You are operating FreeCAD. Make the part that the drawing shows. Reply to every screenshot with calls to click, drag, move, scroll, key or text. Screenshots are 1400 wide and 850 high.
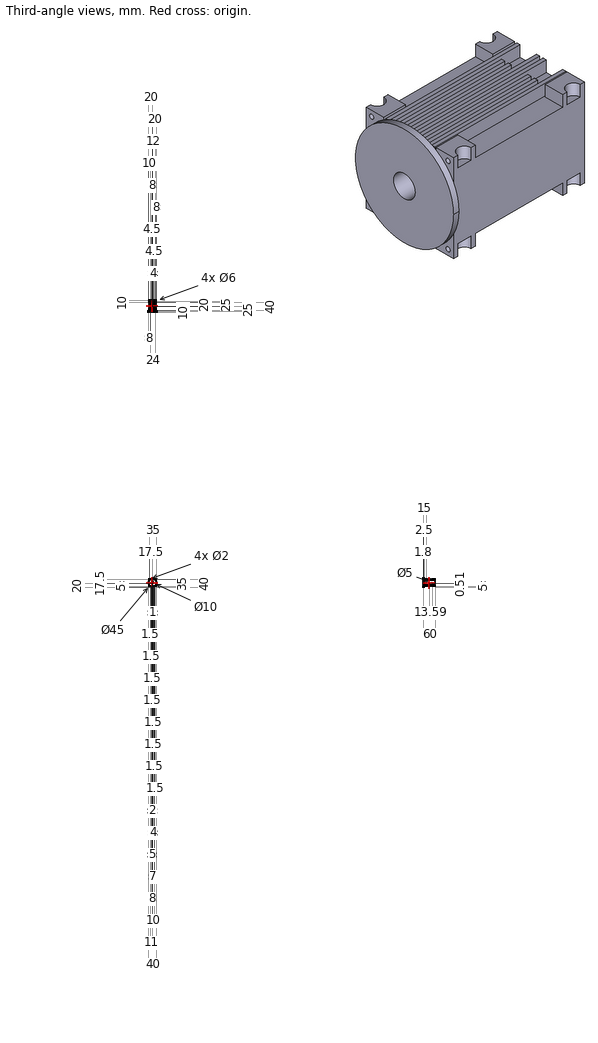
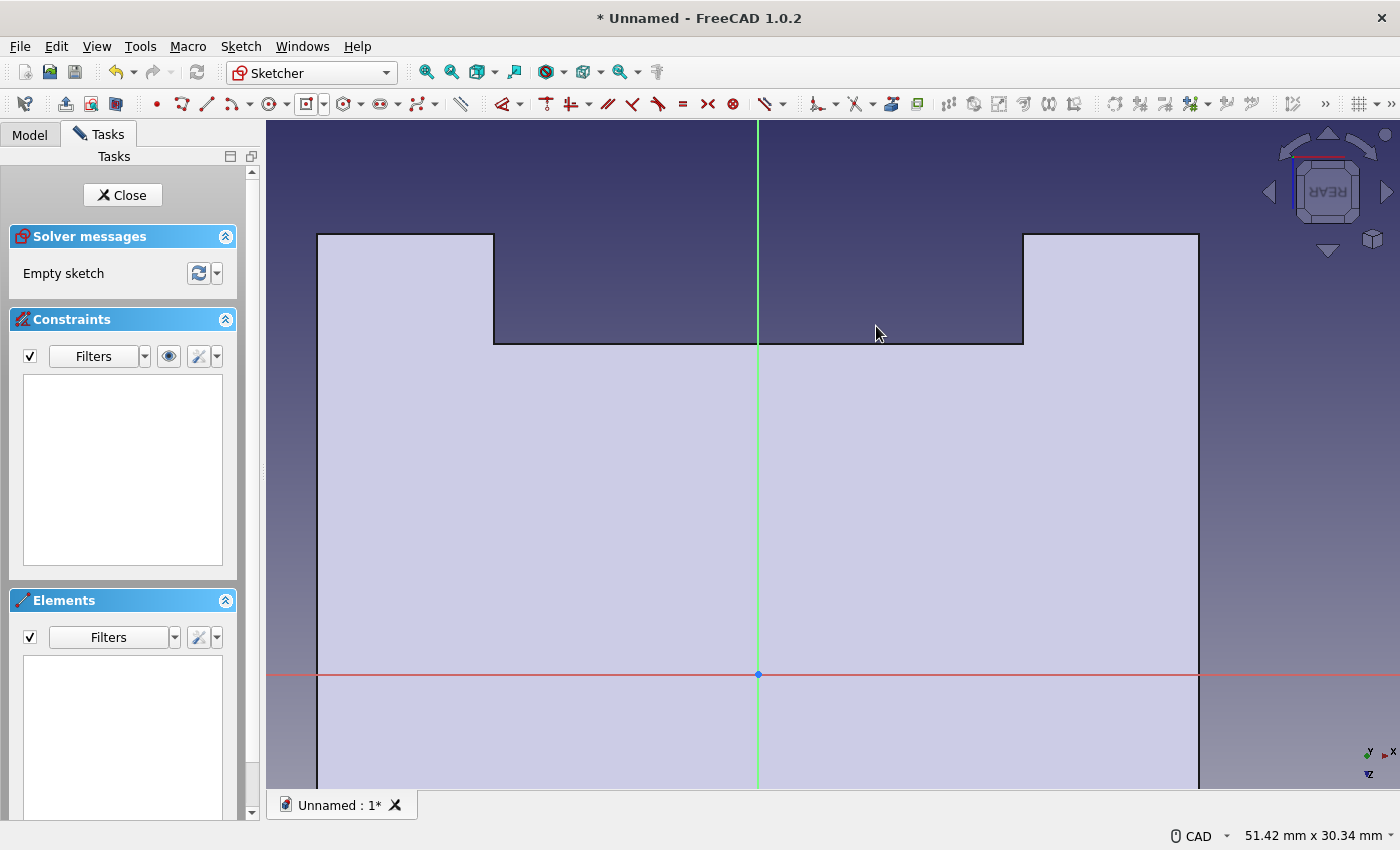
click(324, 104)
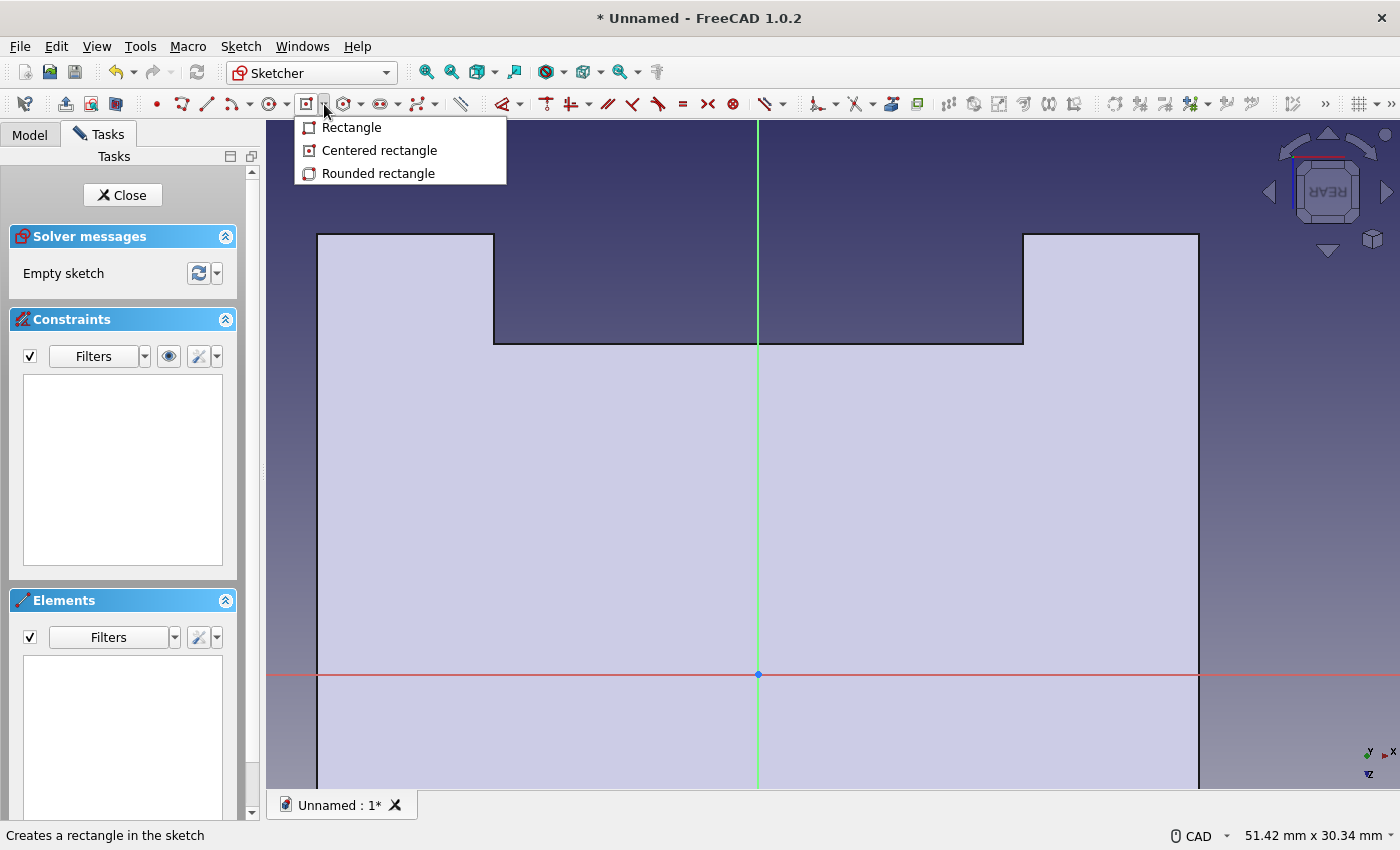
click(400, 128)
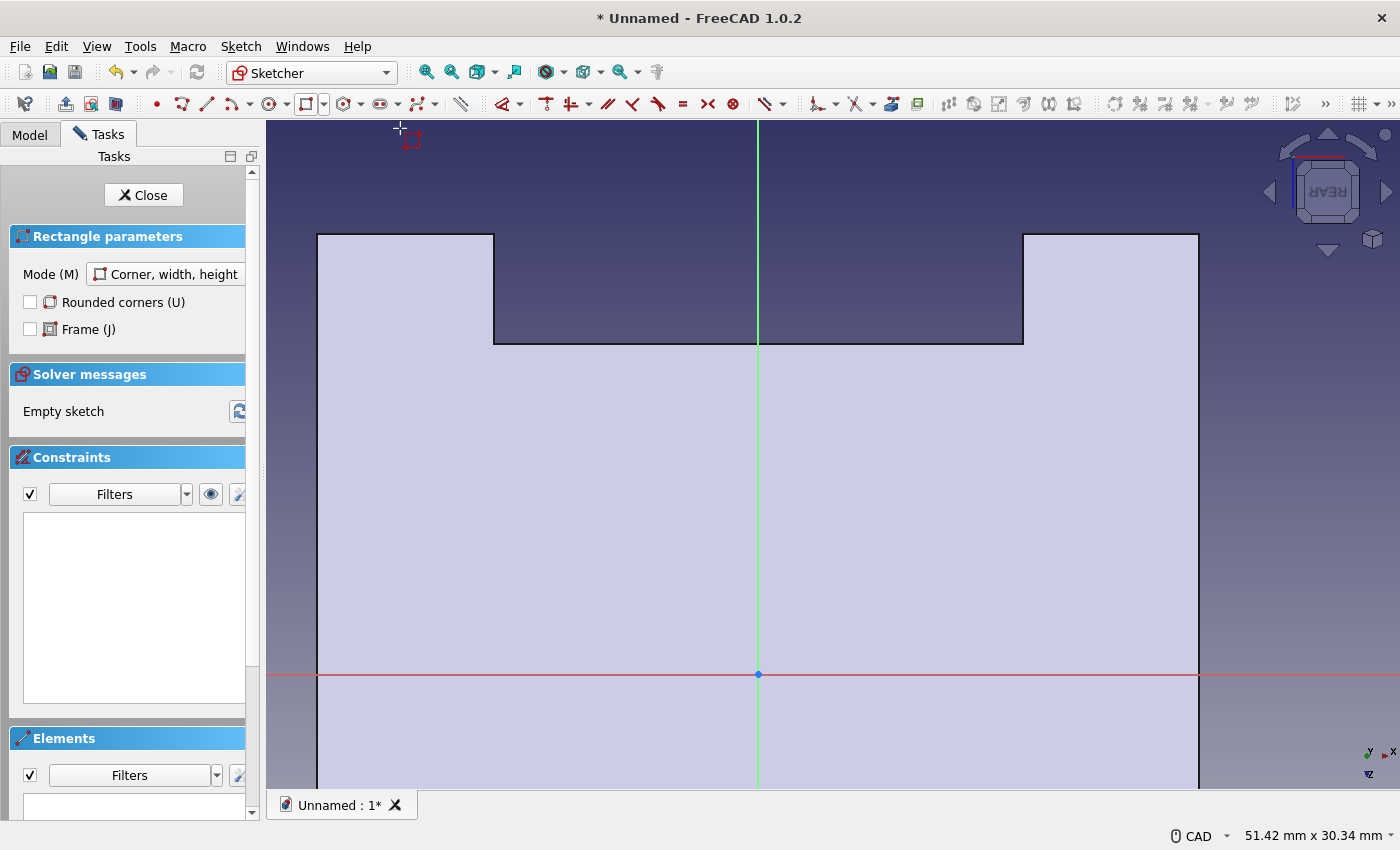
click(516, 234)
click(549, 344)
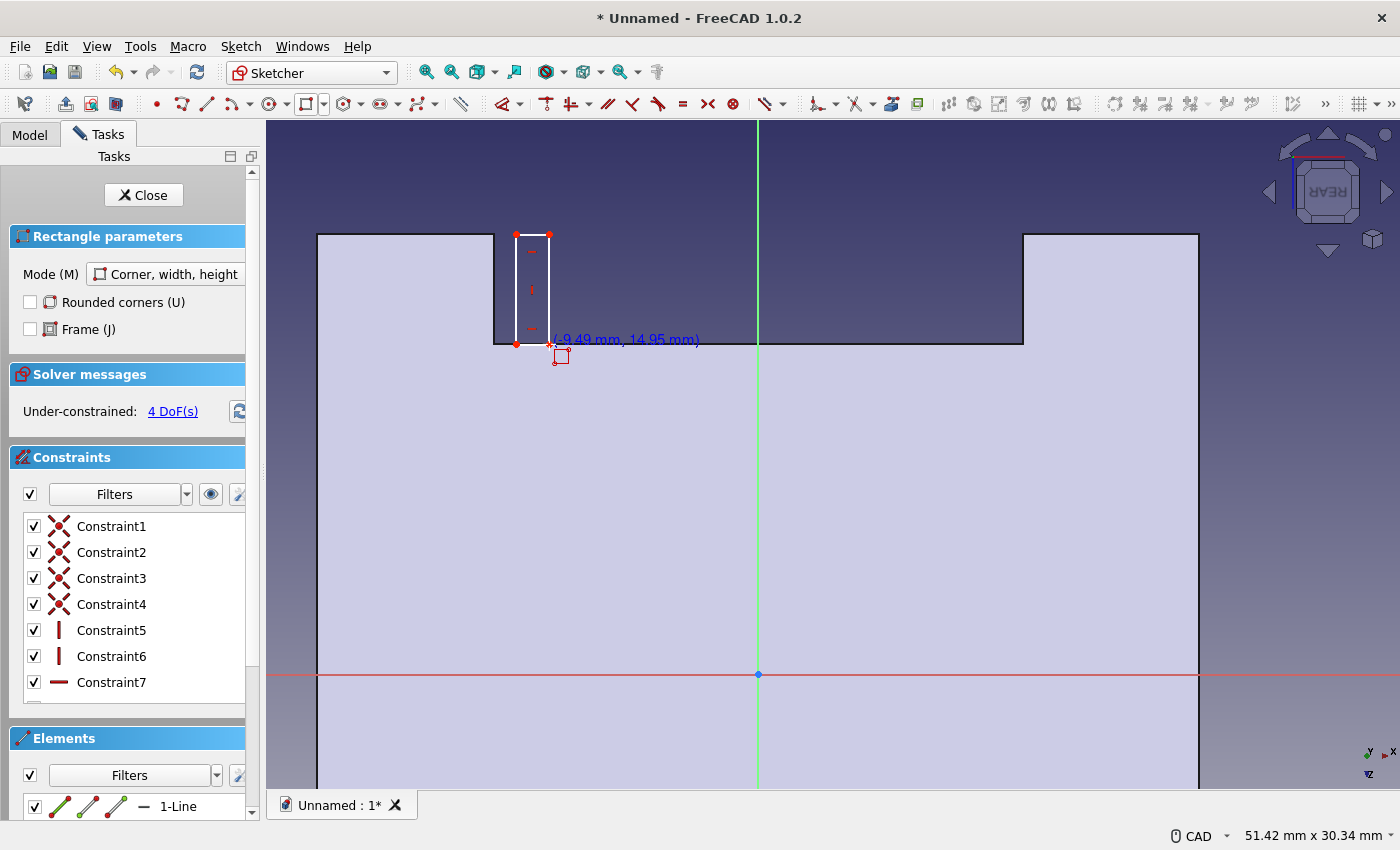
click(582, 234)
click(615, 344)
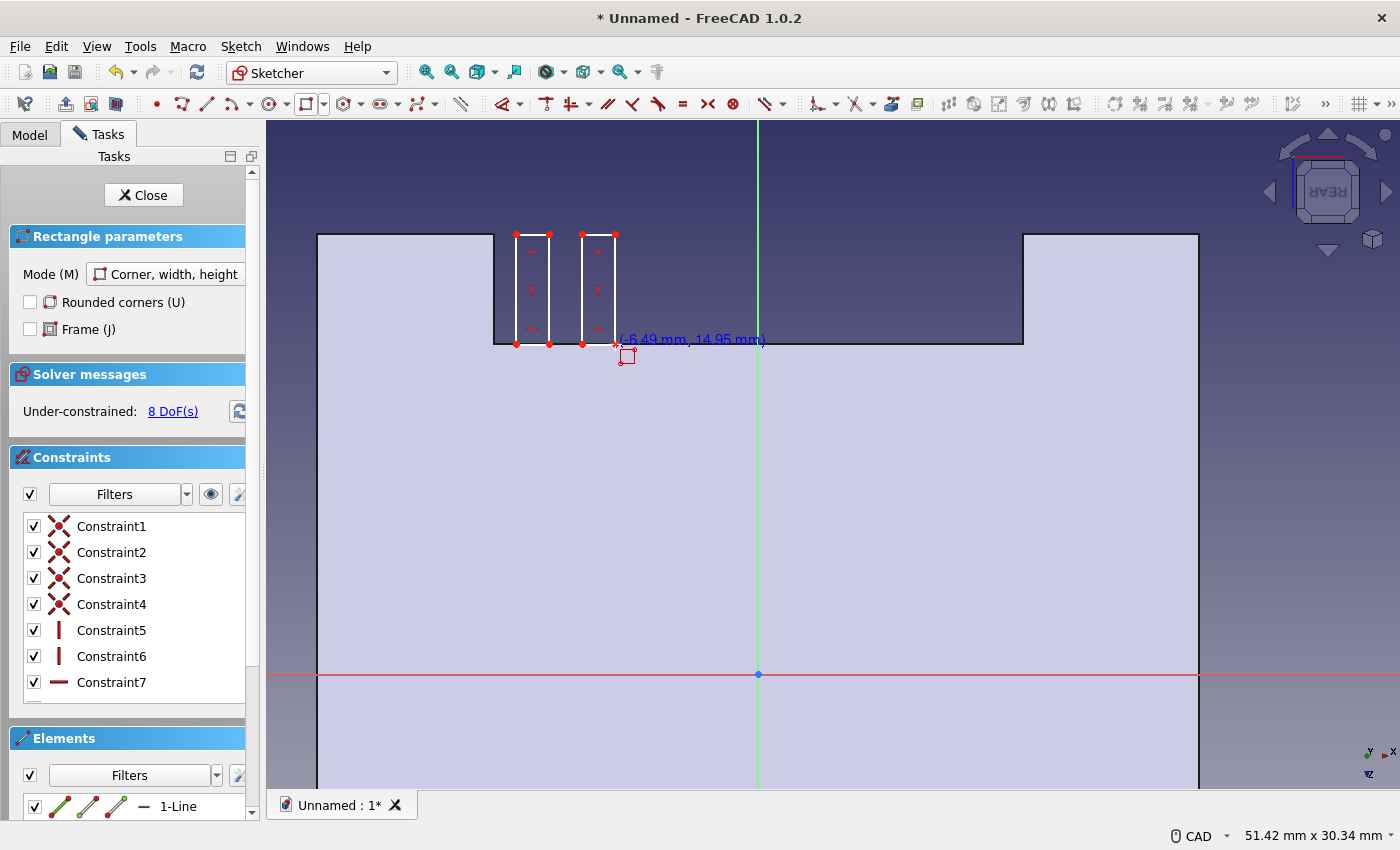
click(648, 234)
click(681, 344)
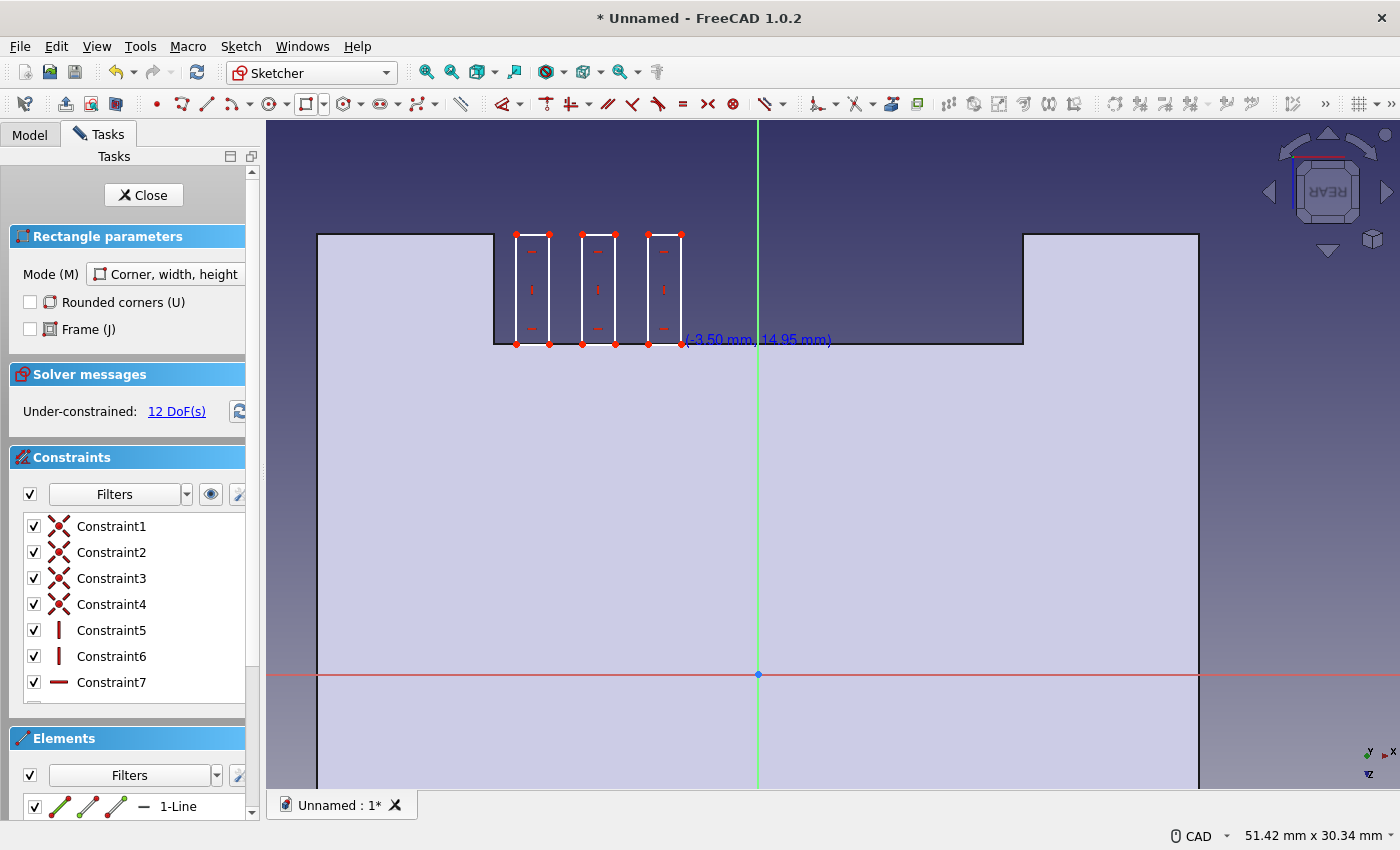
click(714, 234)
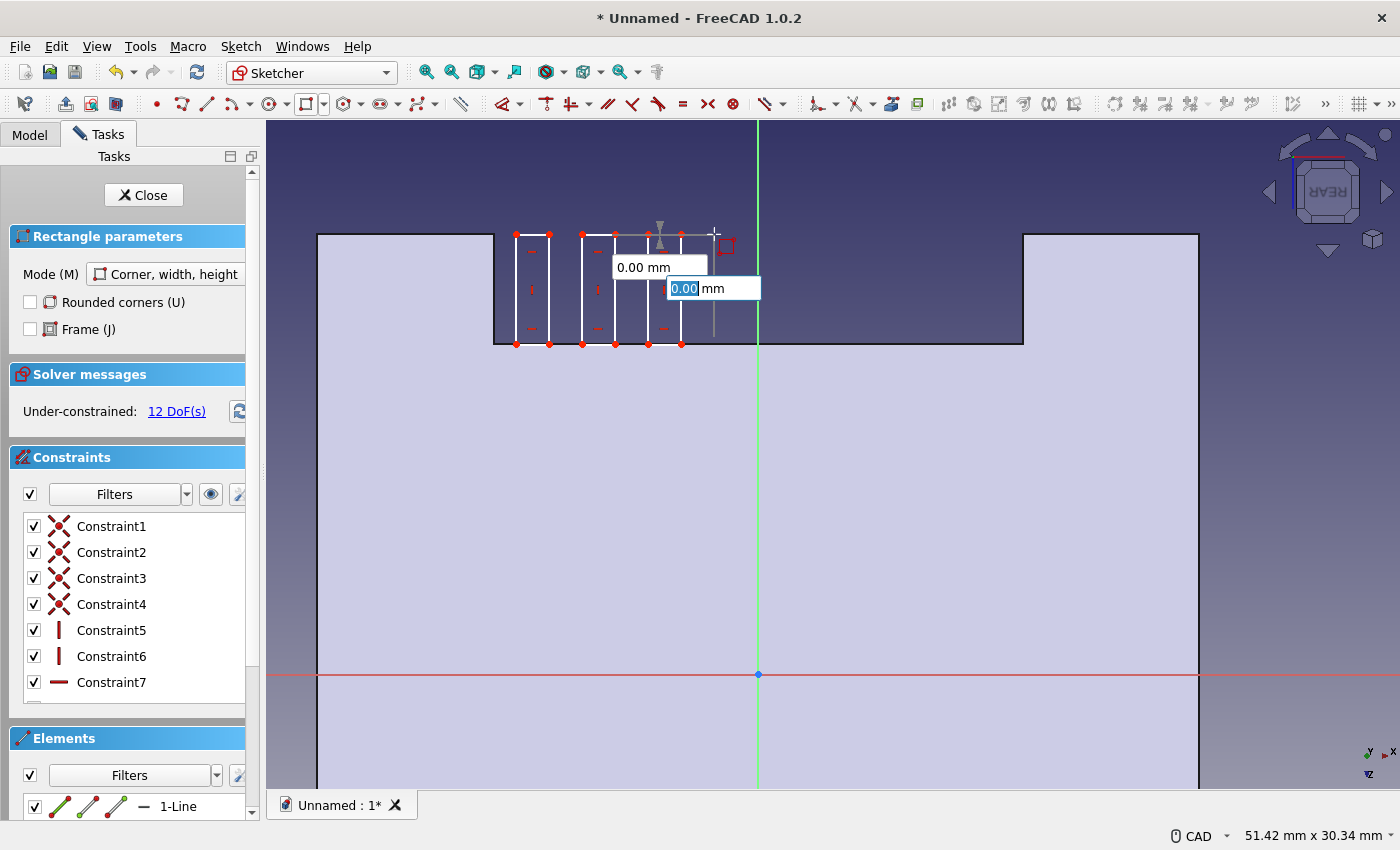
scroll(747, 344, up, 2)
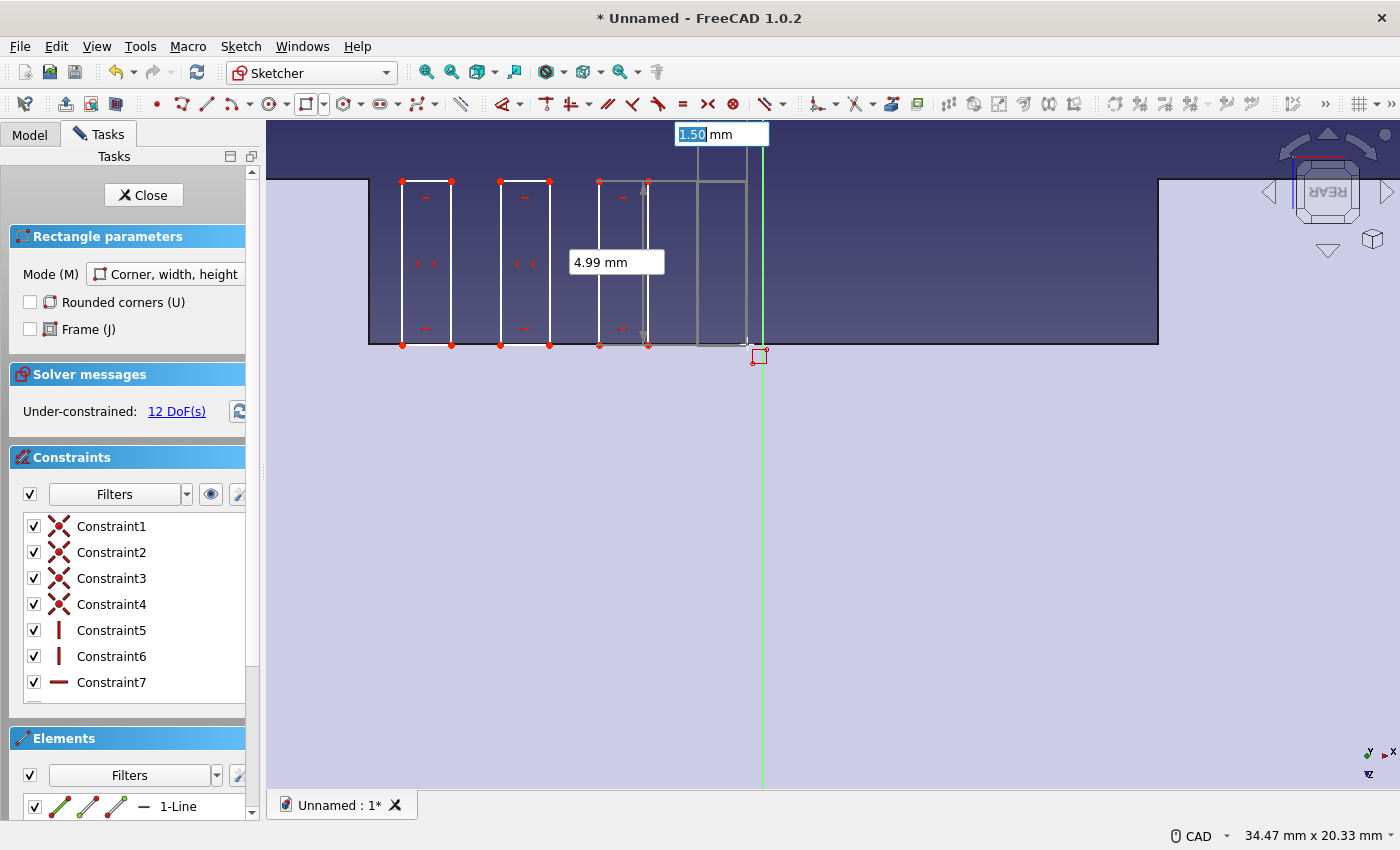
click(747, 344)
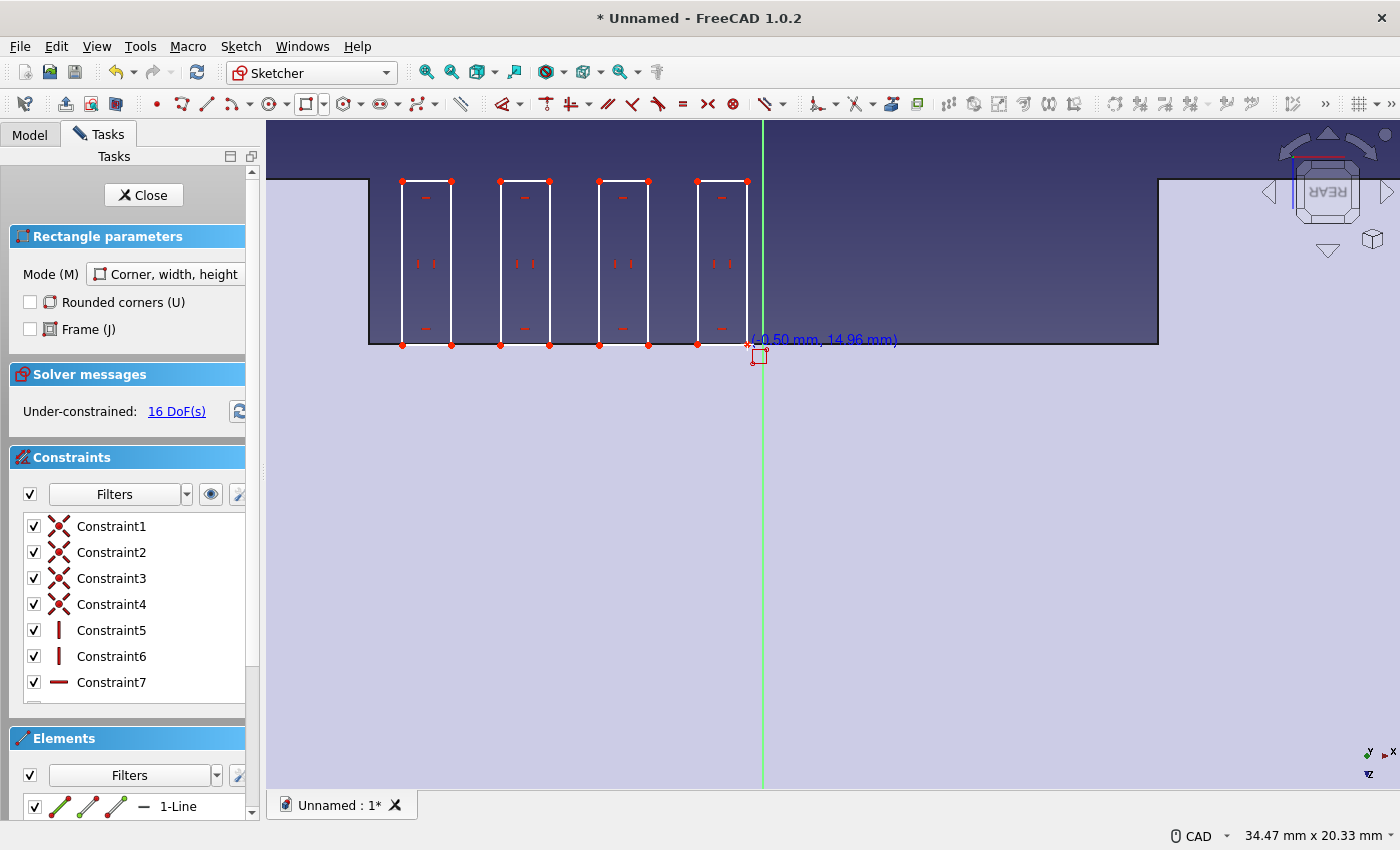
click(796, 179)
click(846, 344)